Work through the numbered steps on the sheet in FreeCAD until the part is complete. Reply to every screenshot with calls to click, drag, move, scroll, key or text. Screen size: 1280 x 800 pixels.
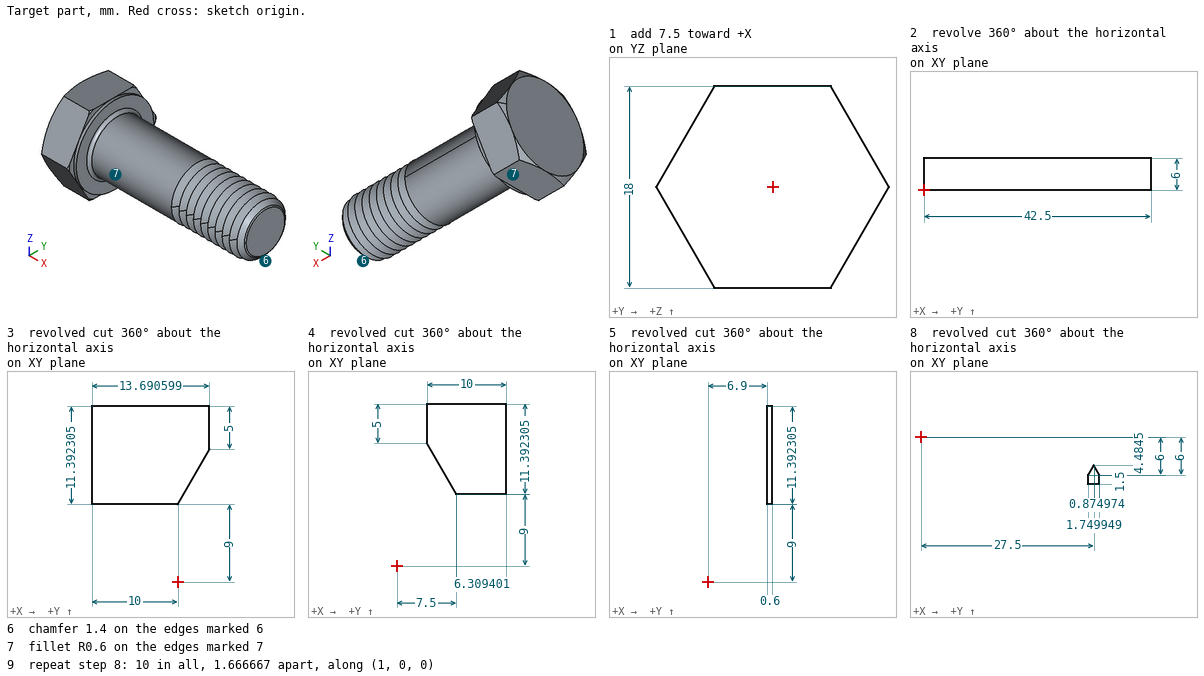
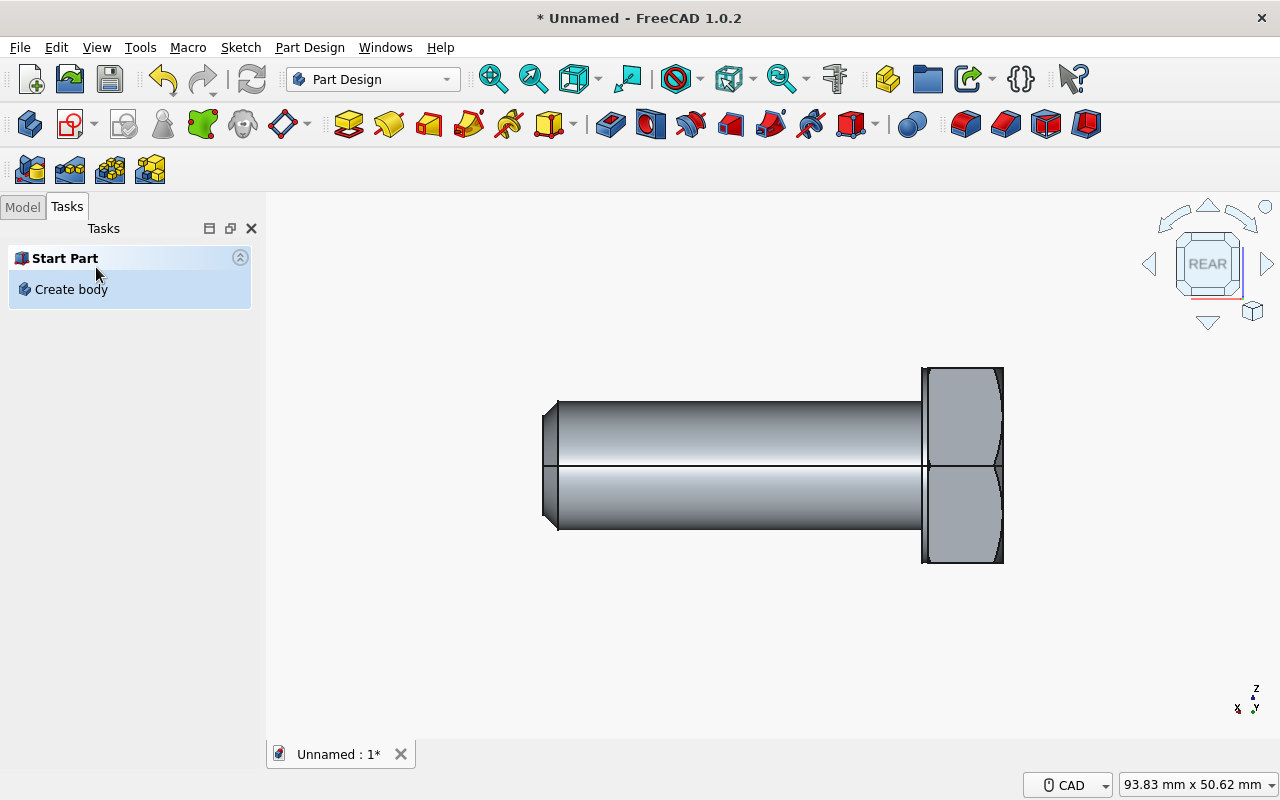
key(6)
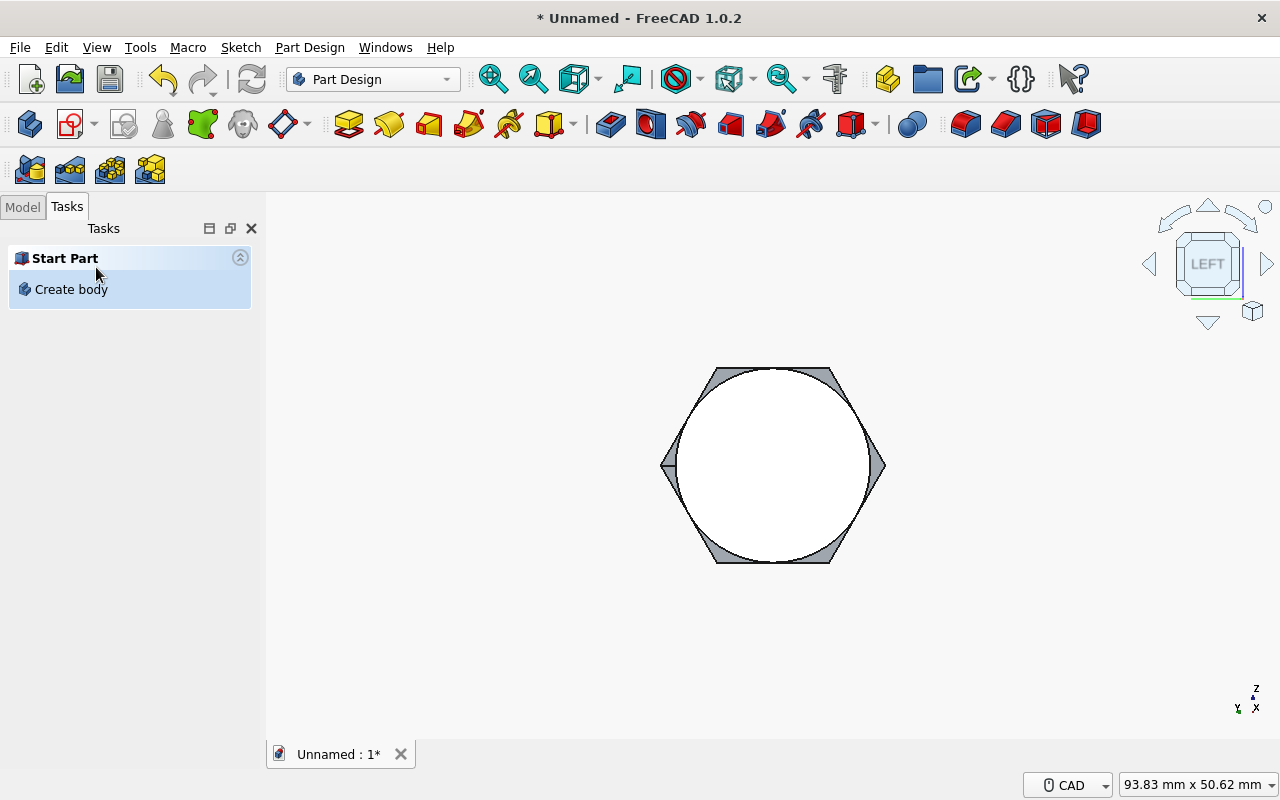
key(v)
key(f)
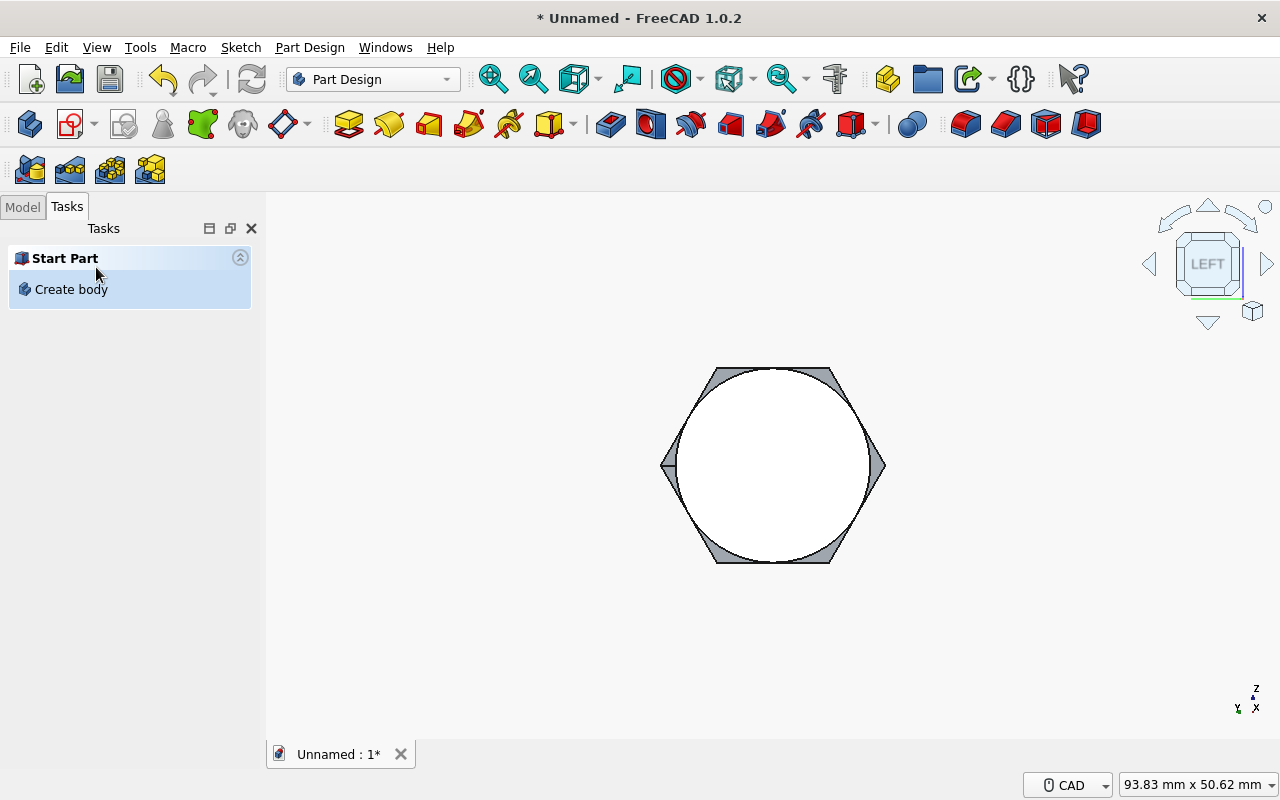
key(v)
key(3)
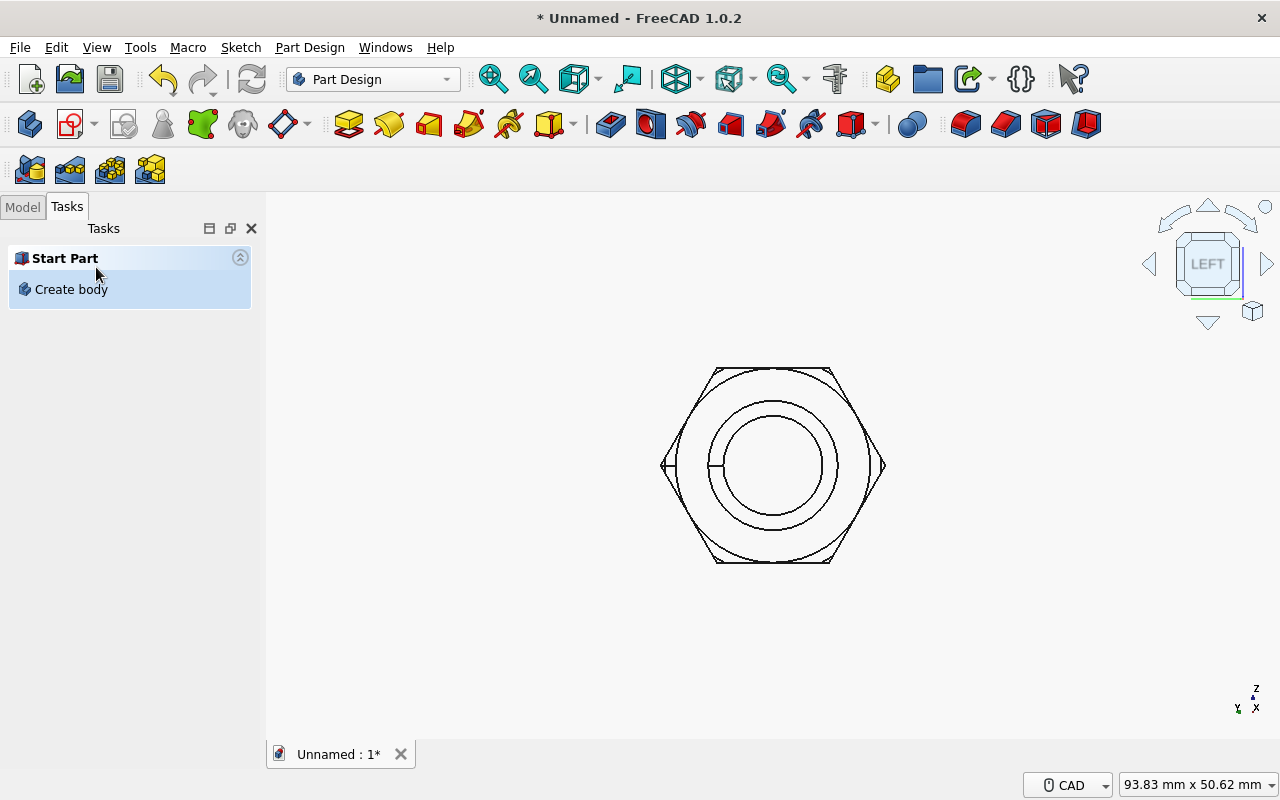
key(0)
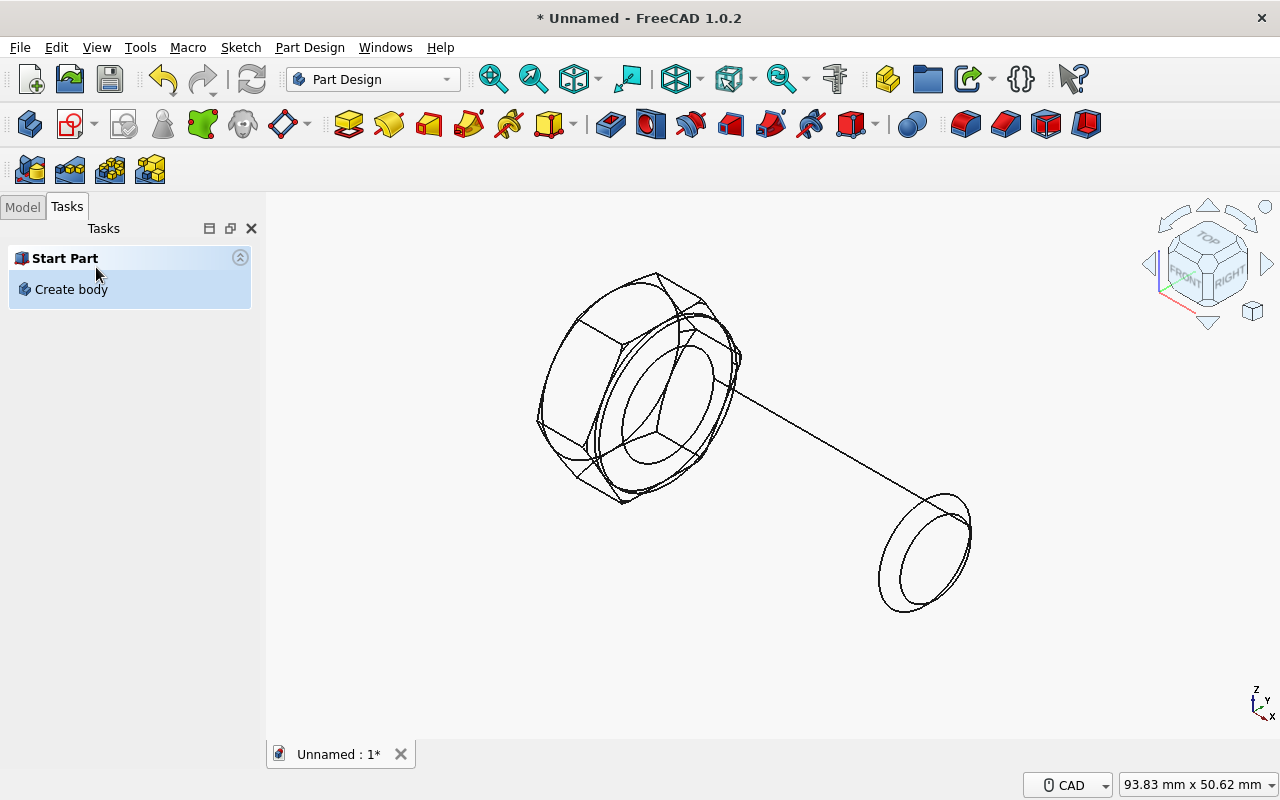
click(622, 430)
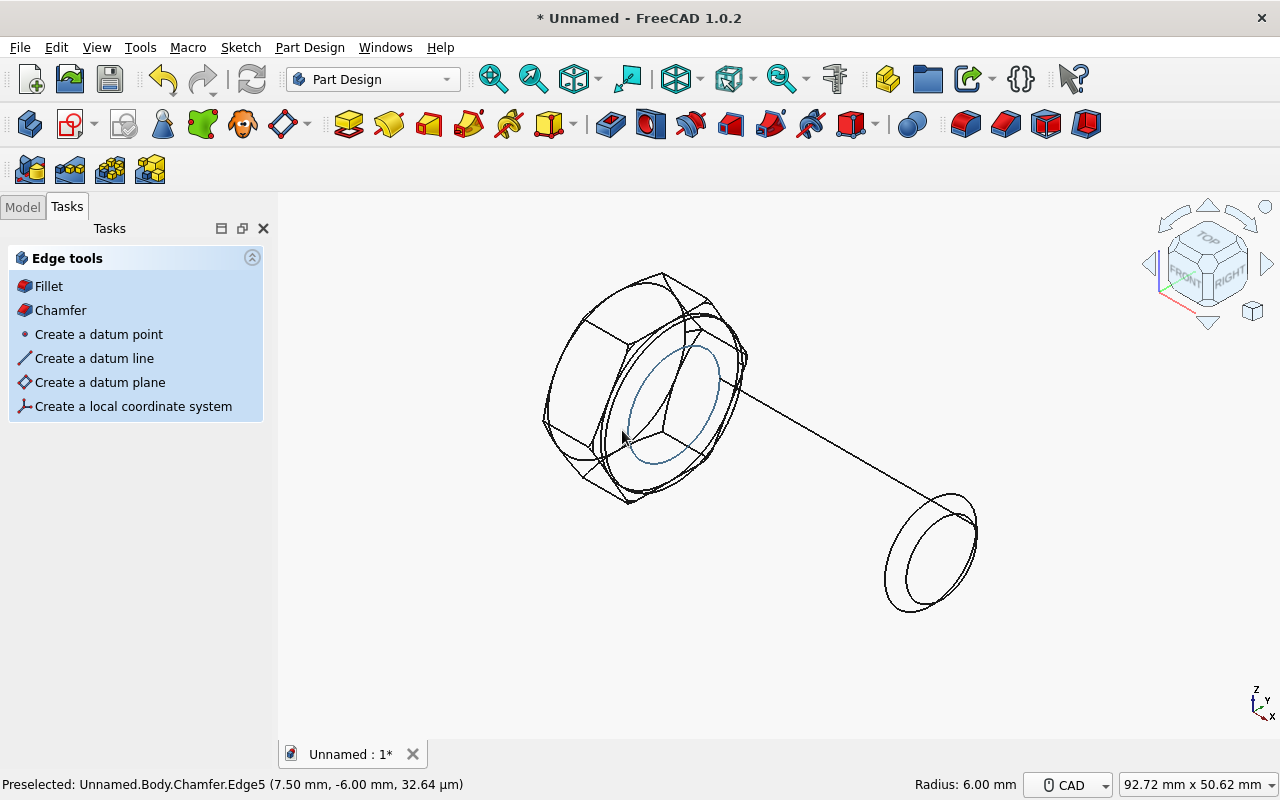
key(v)
key(1)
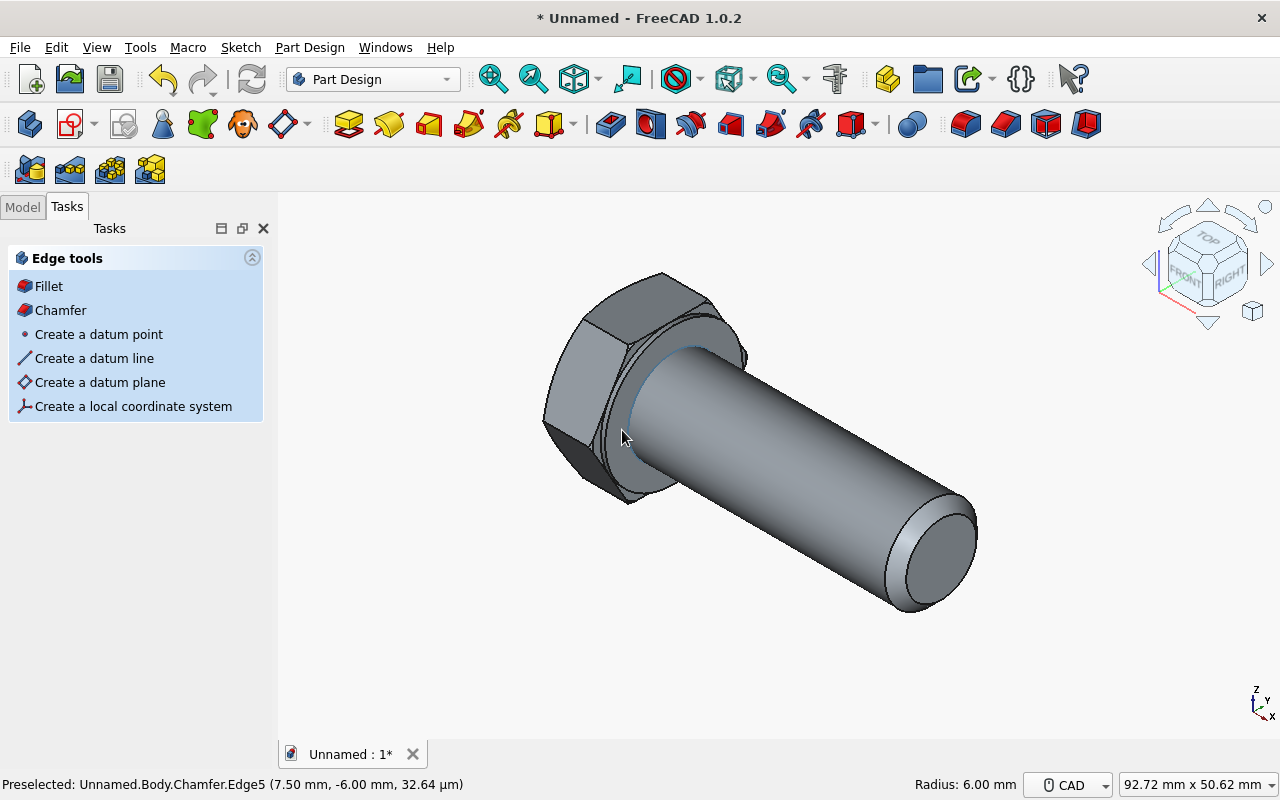
click(966, 124)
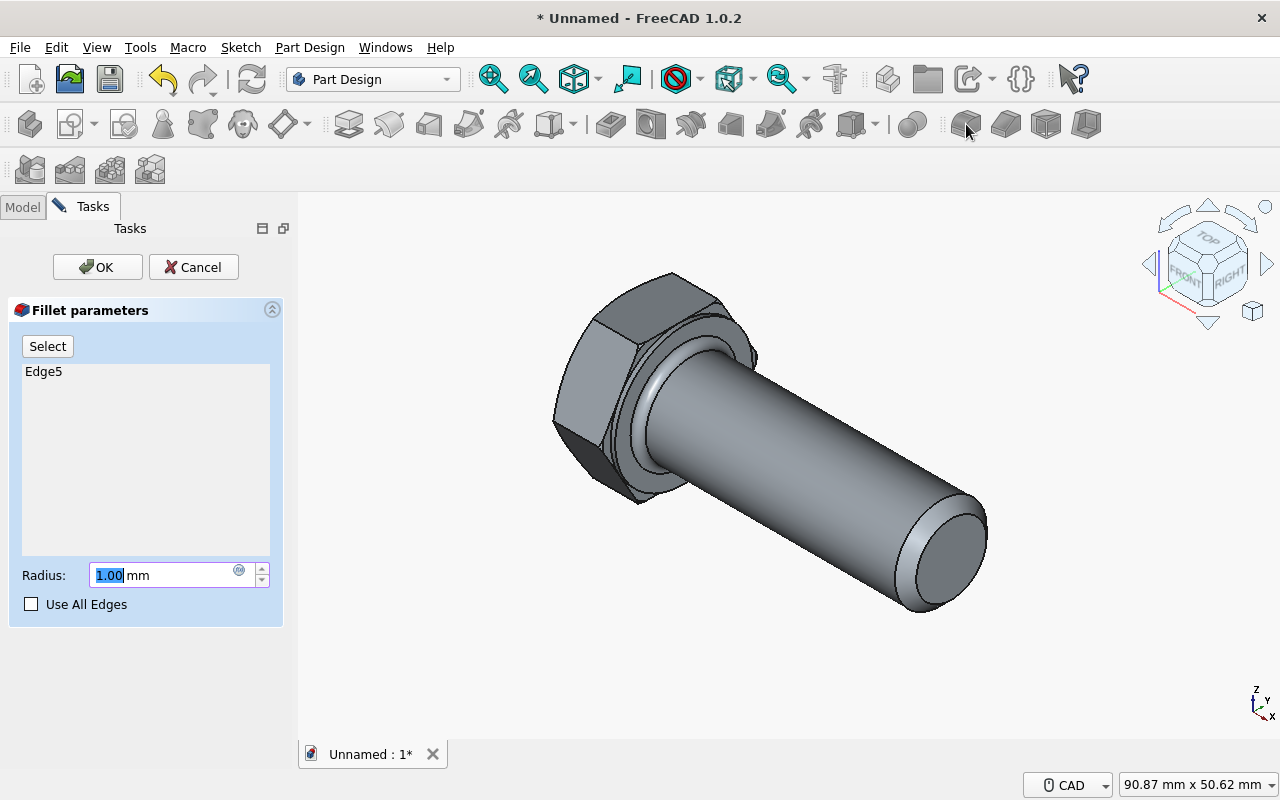
text(0.6)
key(Tab)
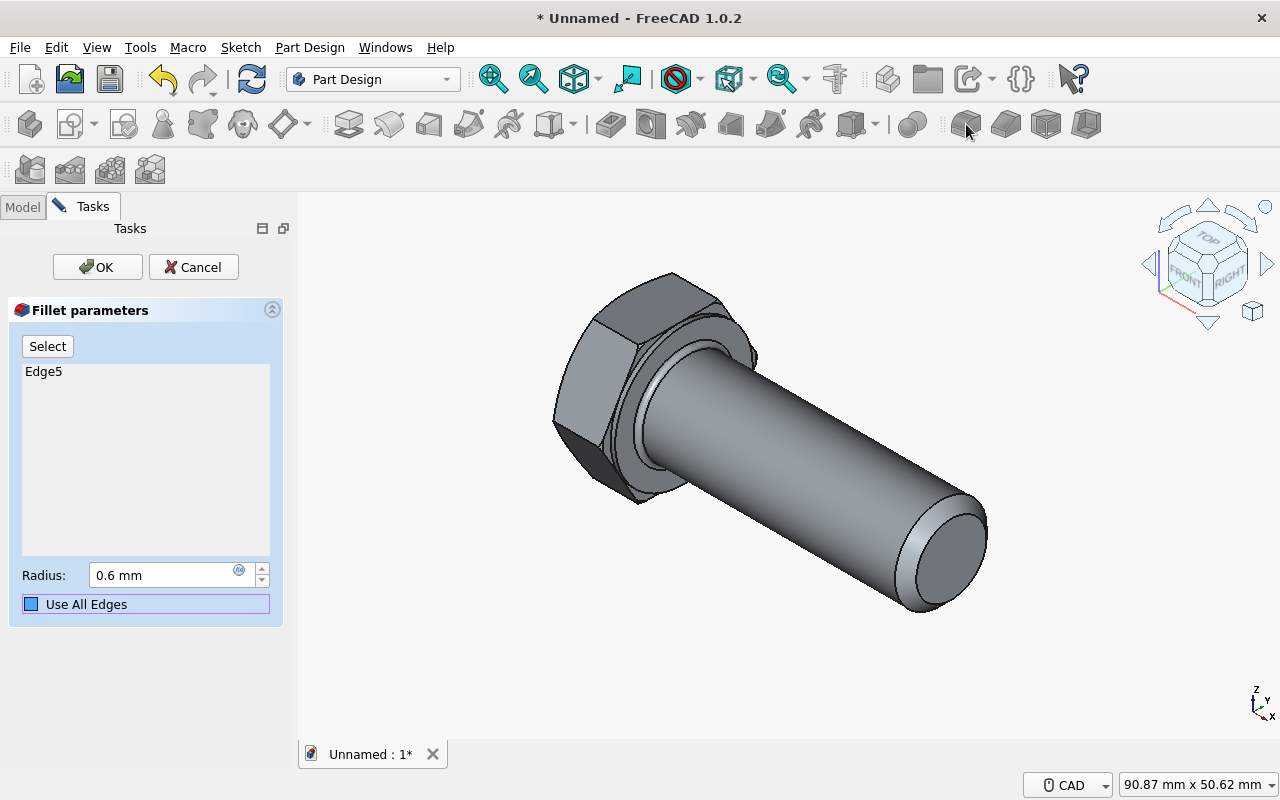
click(98, 267)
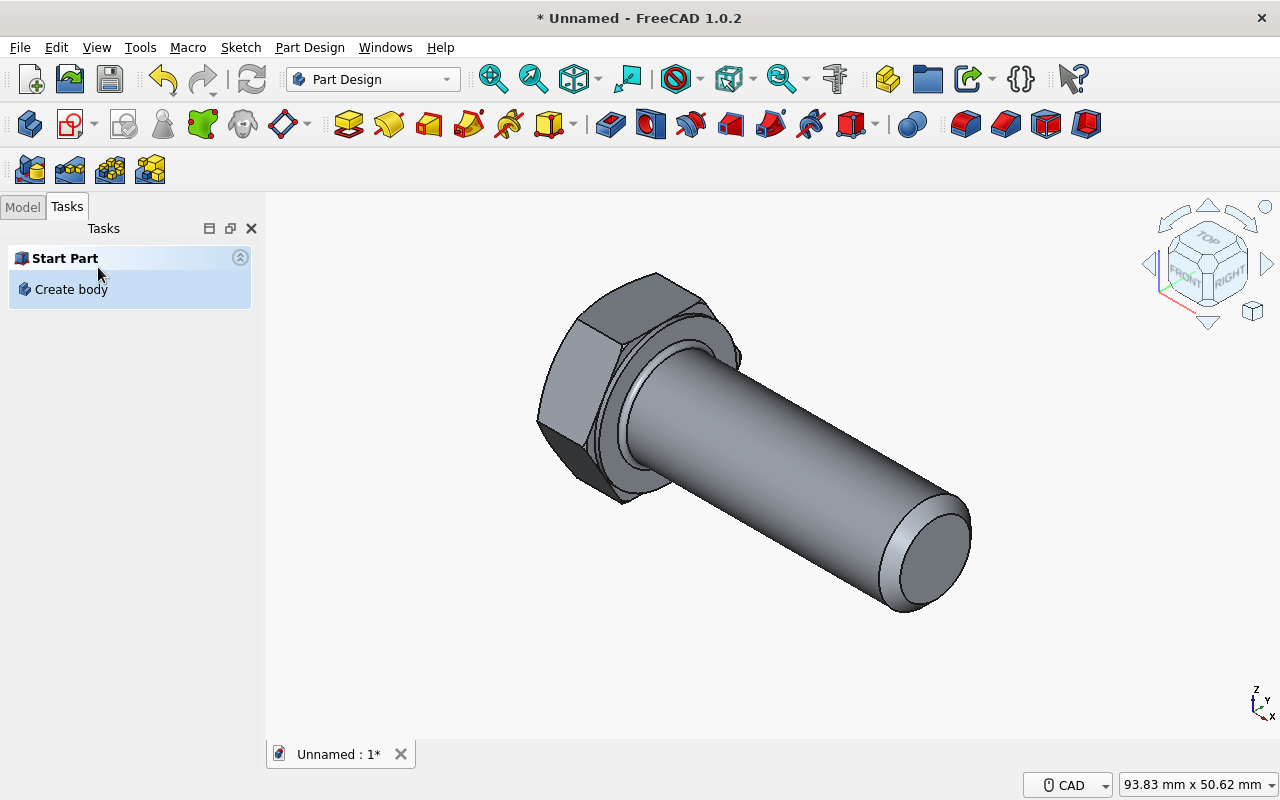
click(70, 124)